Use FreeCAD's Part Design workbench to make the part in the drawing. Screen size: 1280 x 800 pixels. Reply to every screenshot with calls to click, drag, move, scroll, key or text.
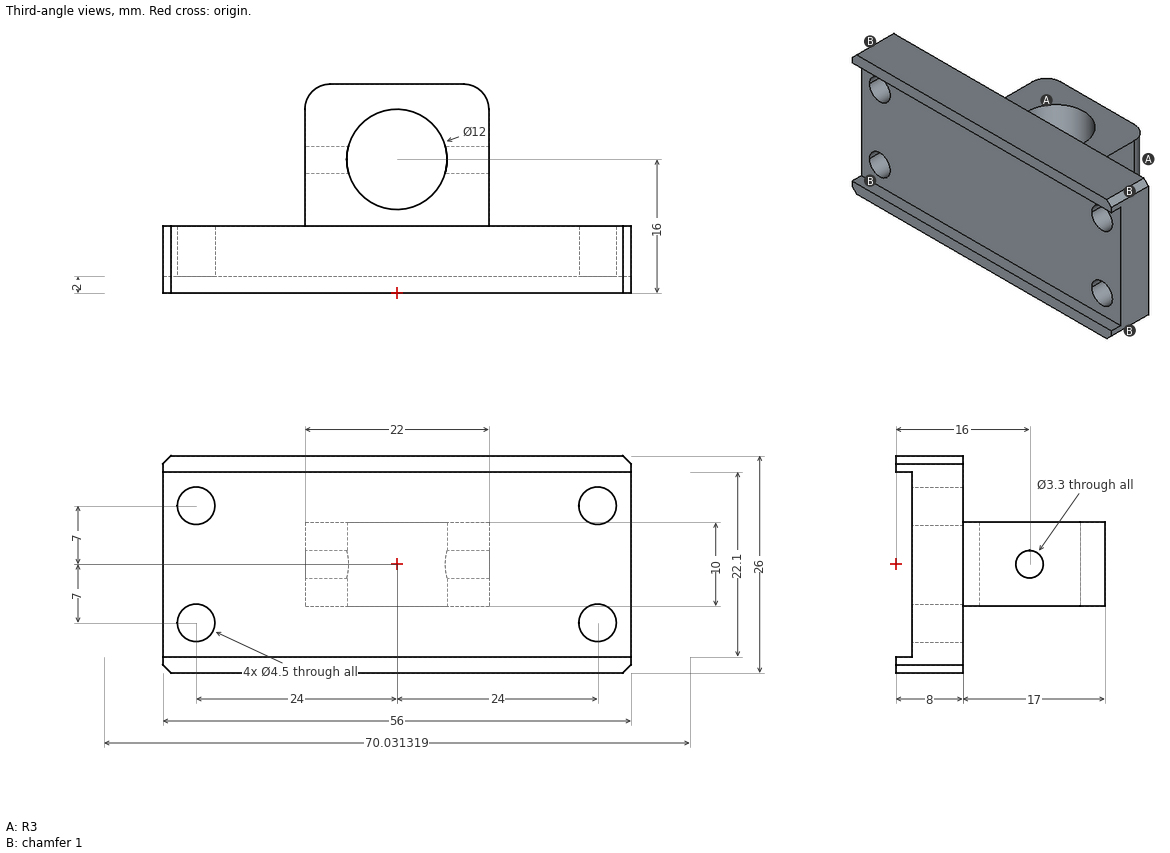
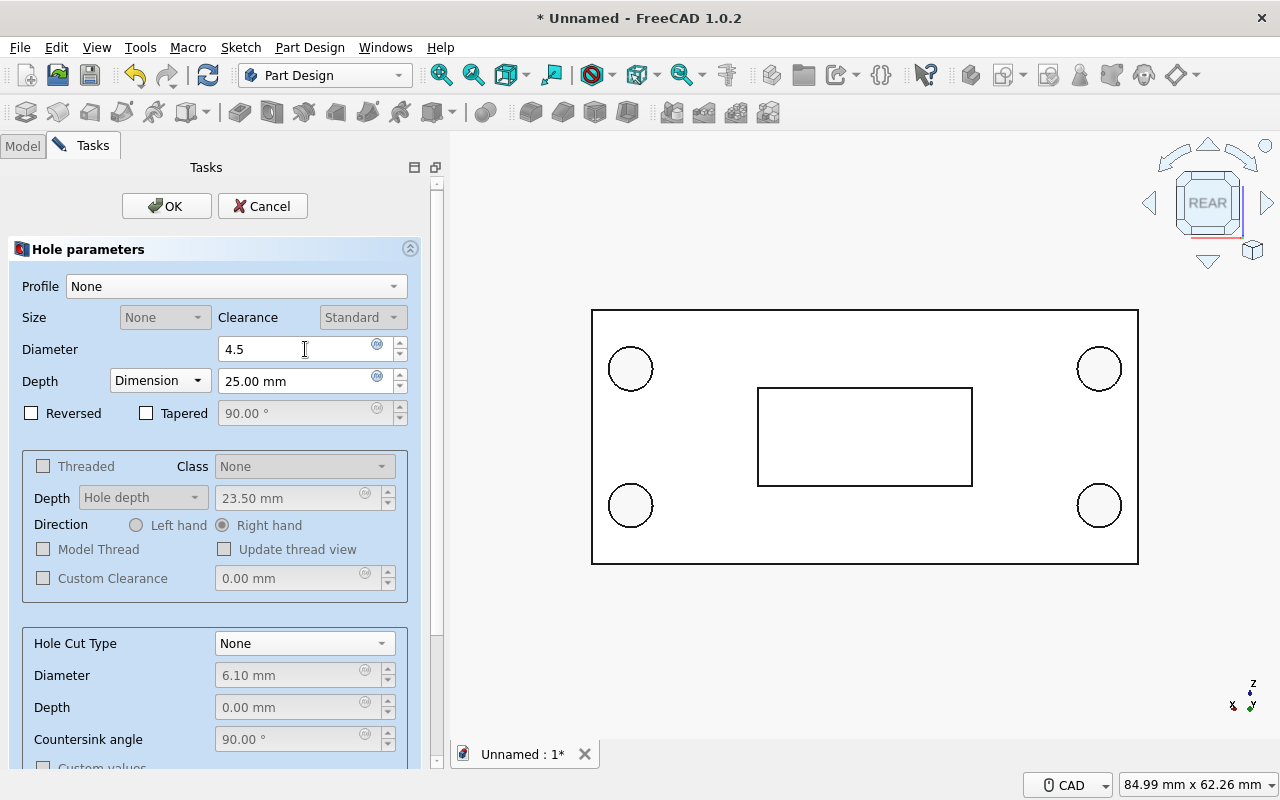
click(161, 380)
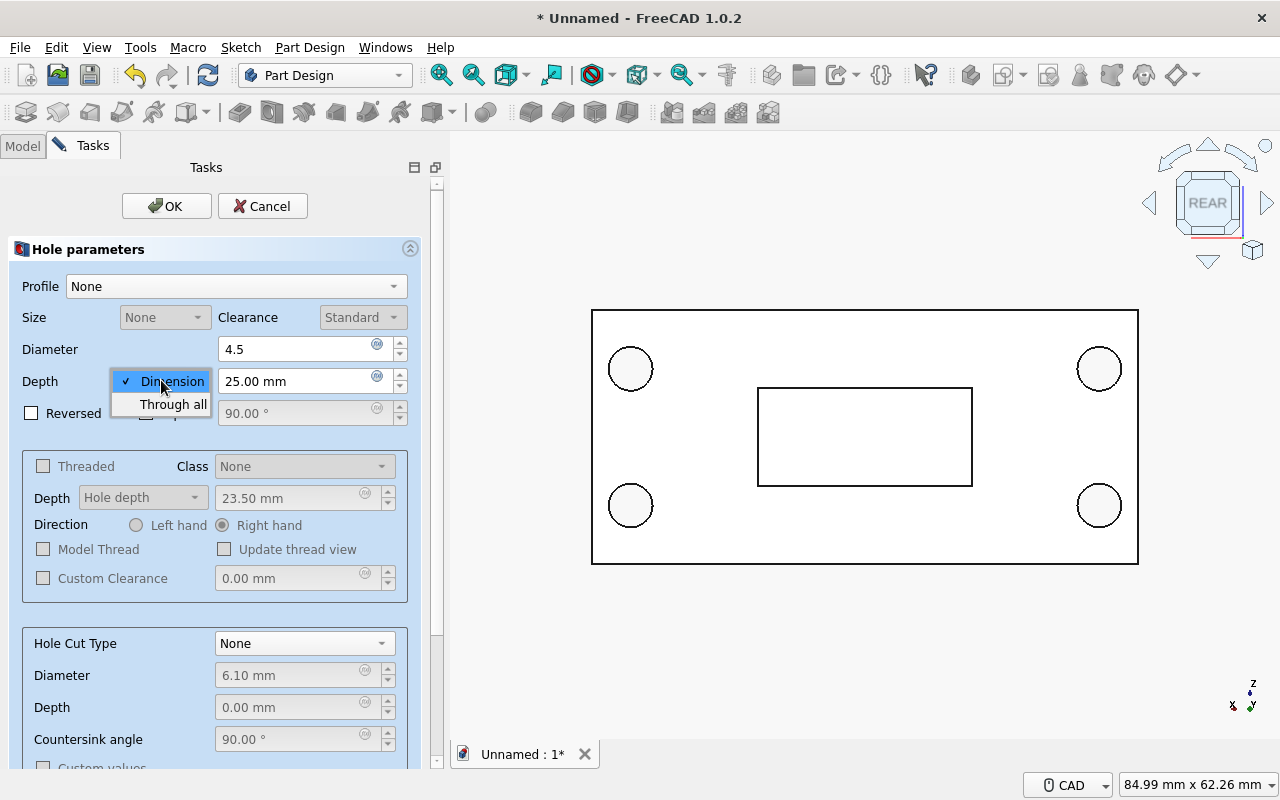
click(160, 404)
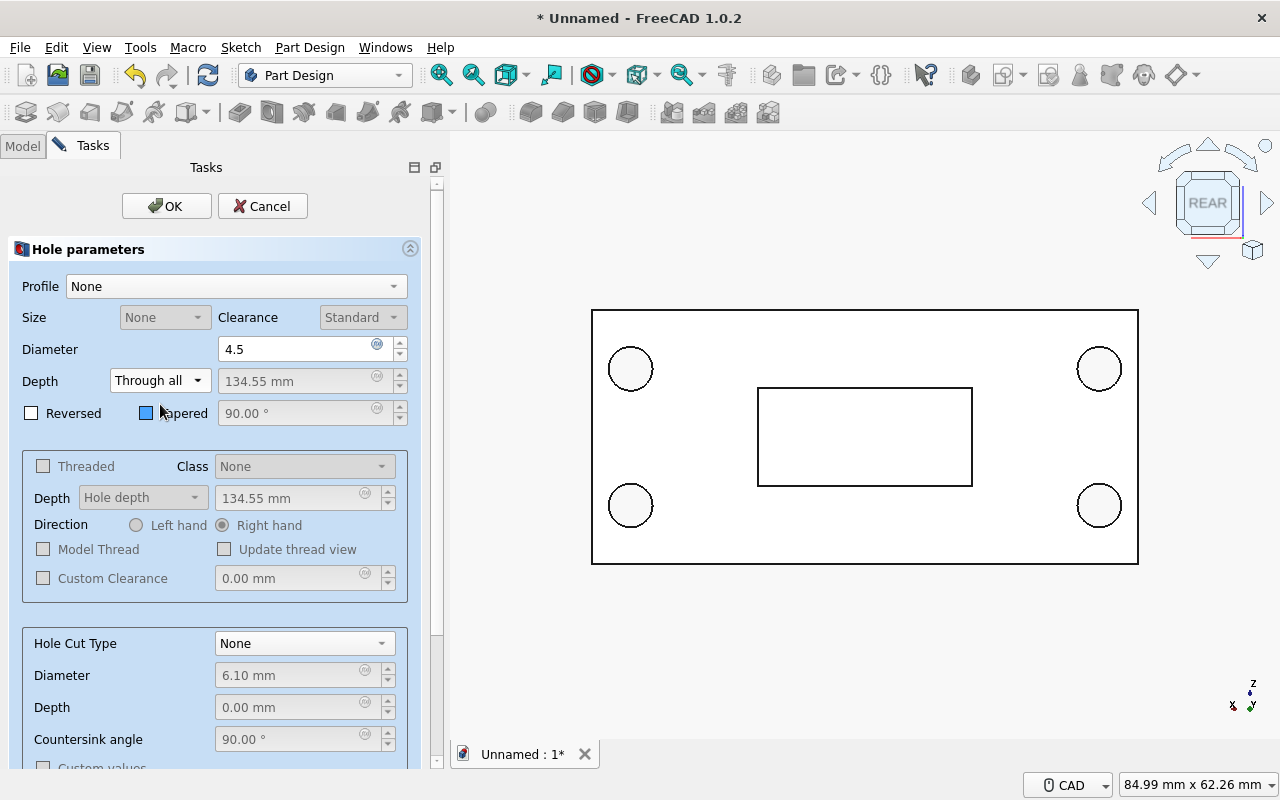
click(167, 206)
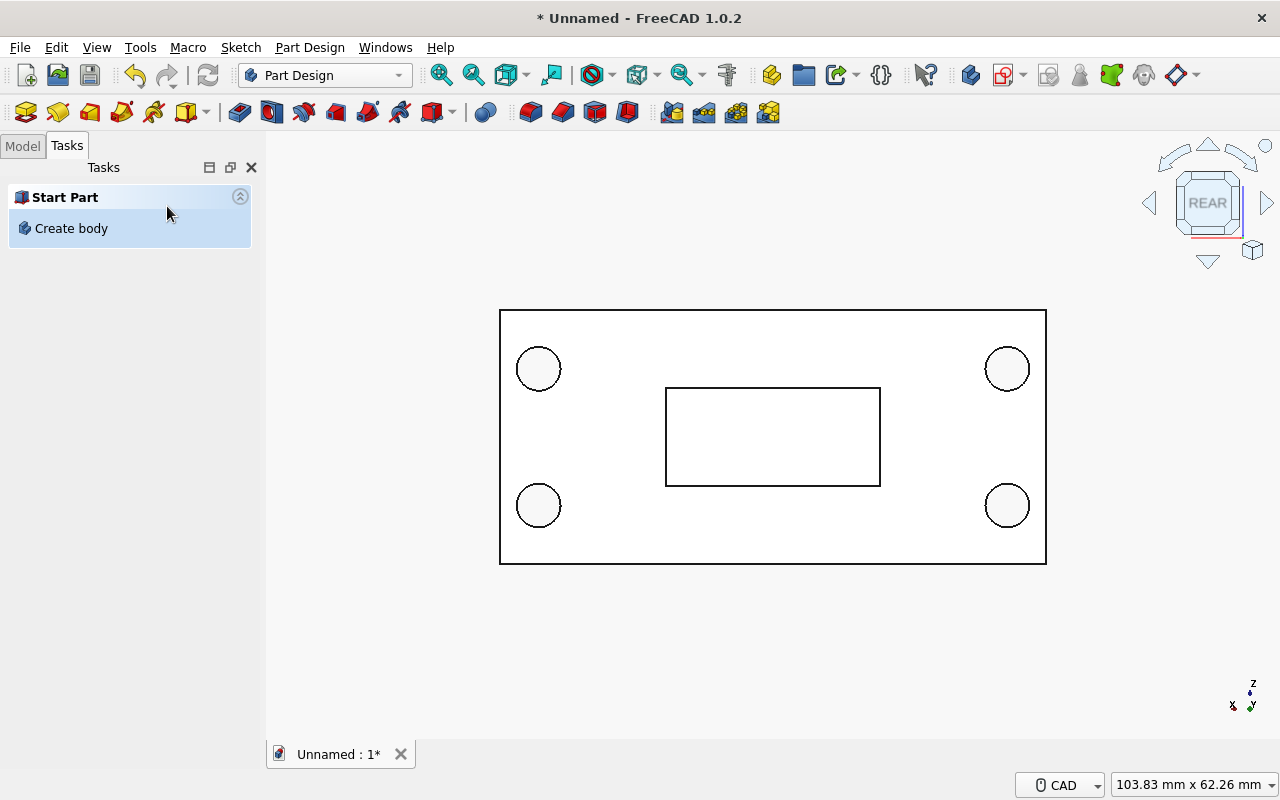
click(880, 436)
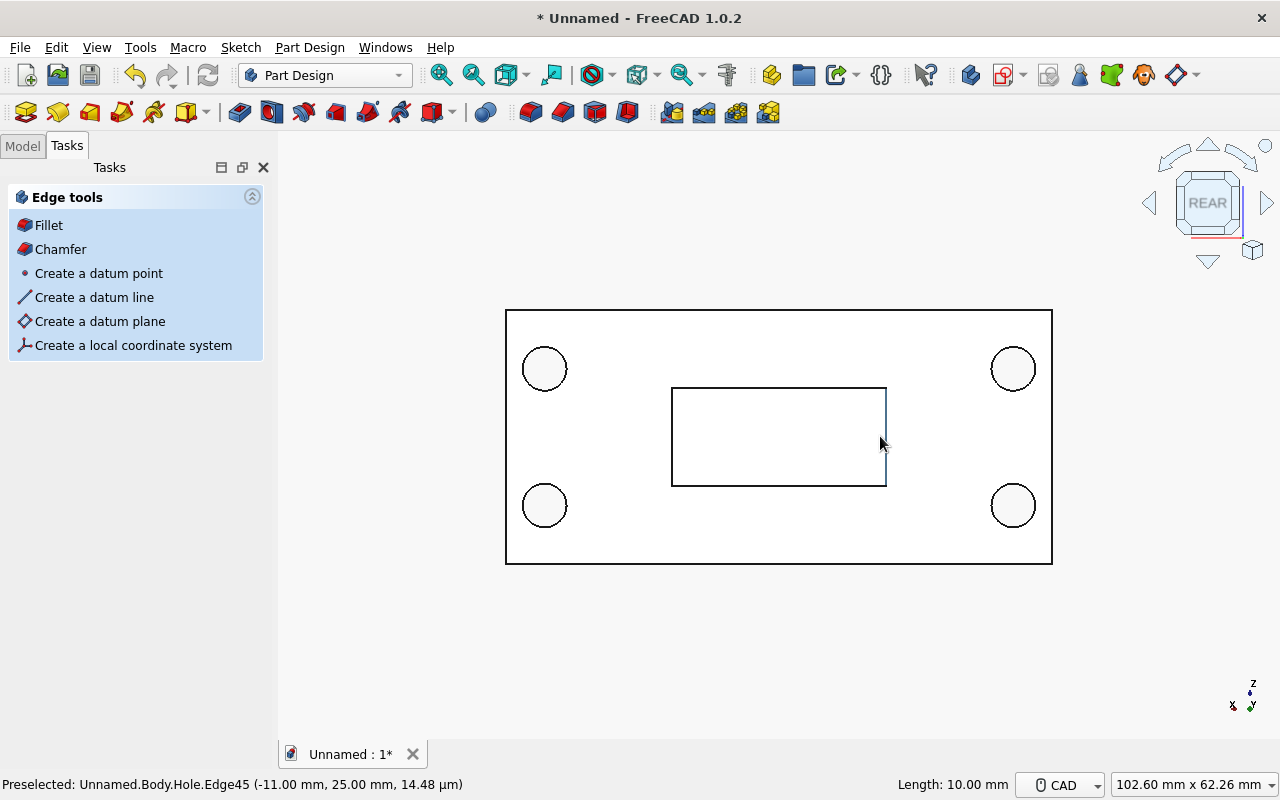
key(0)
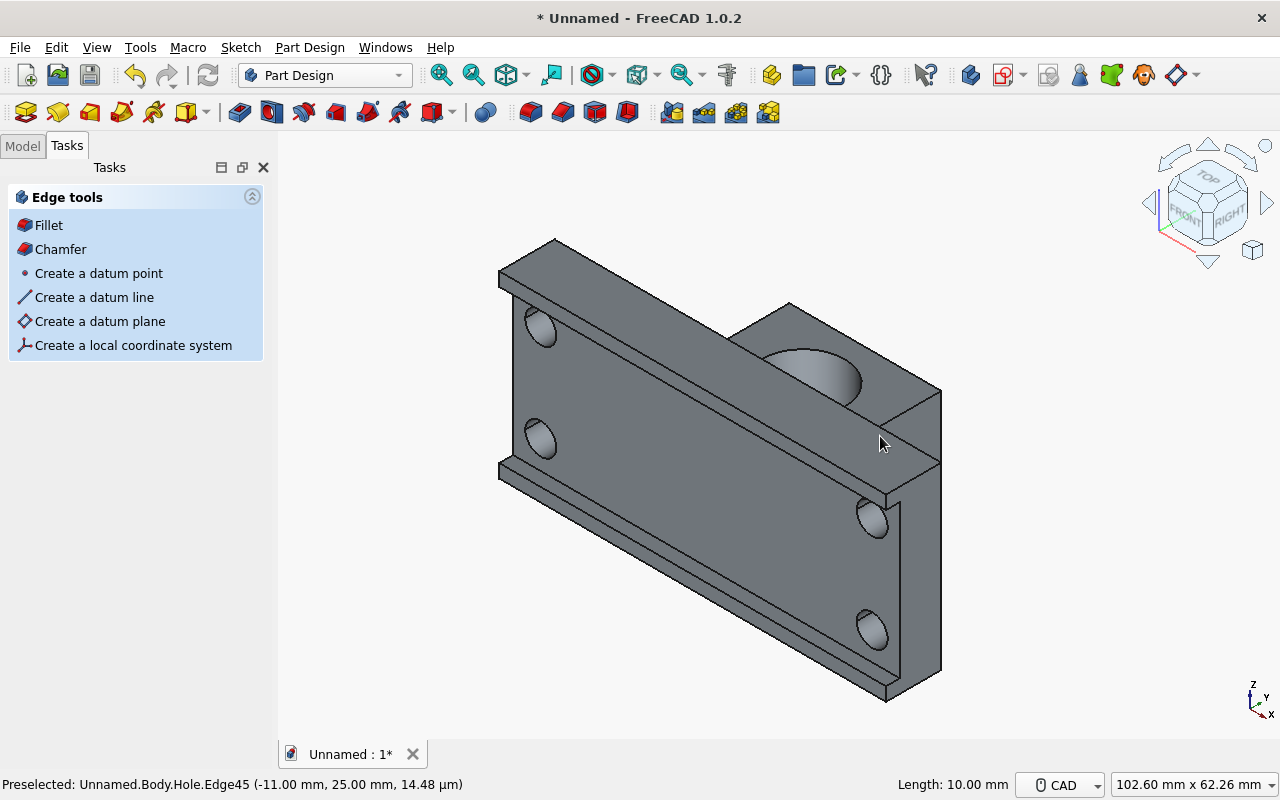
key(2)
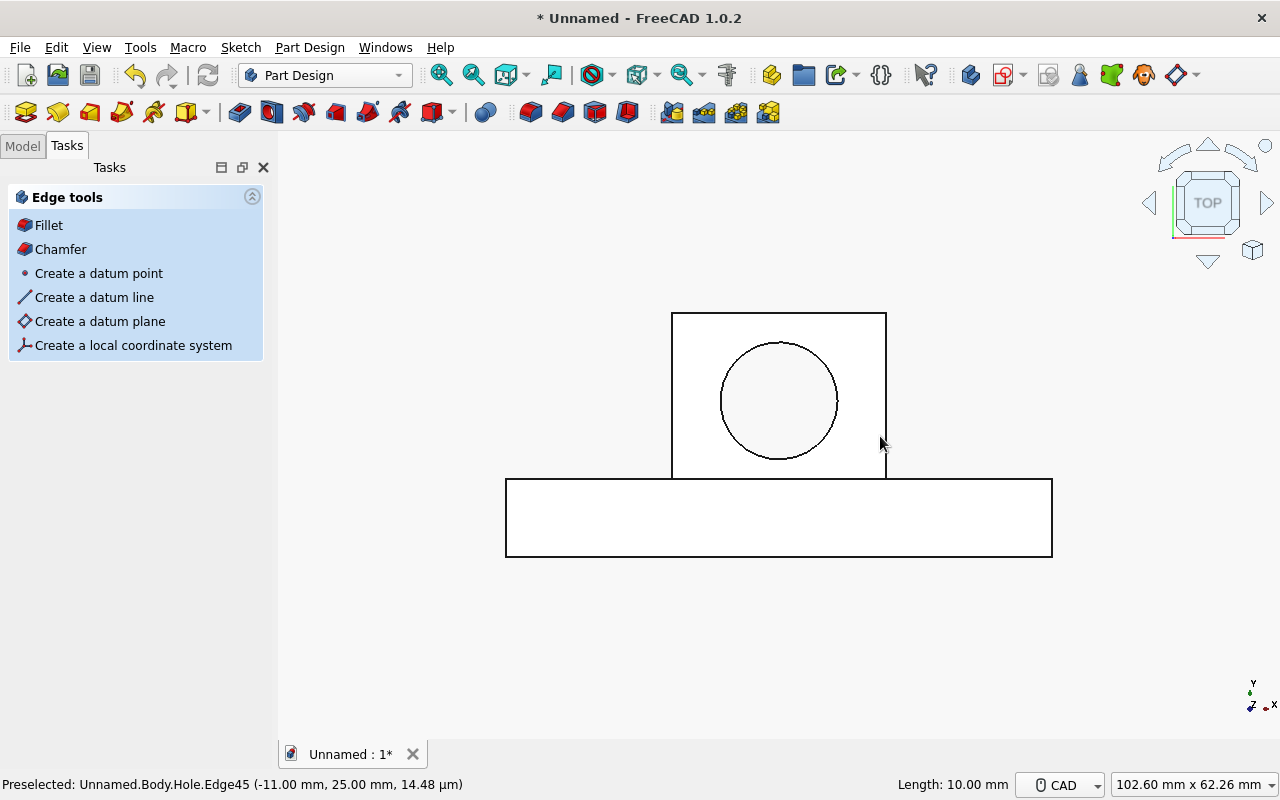
key(1)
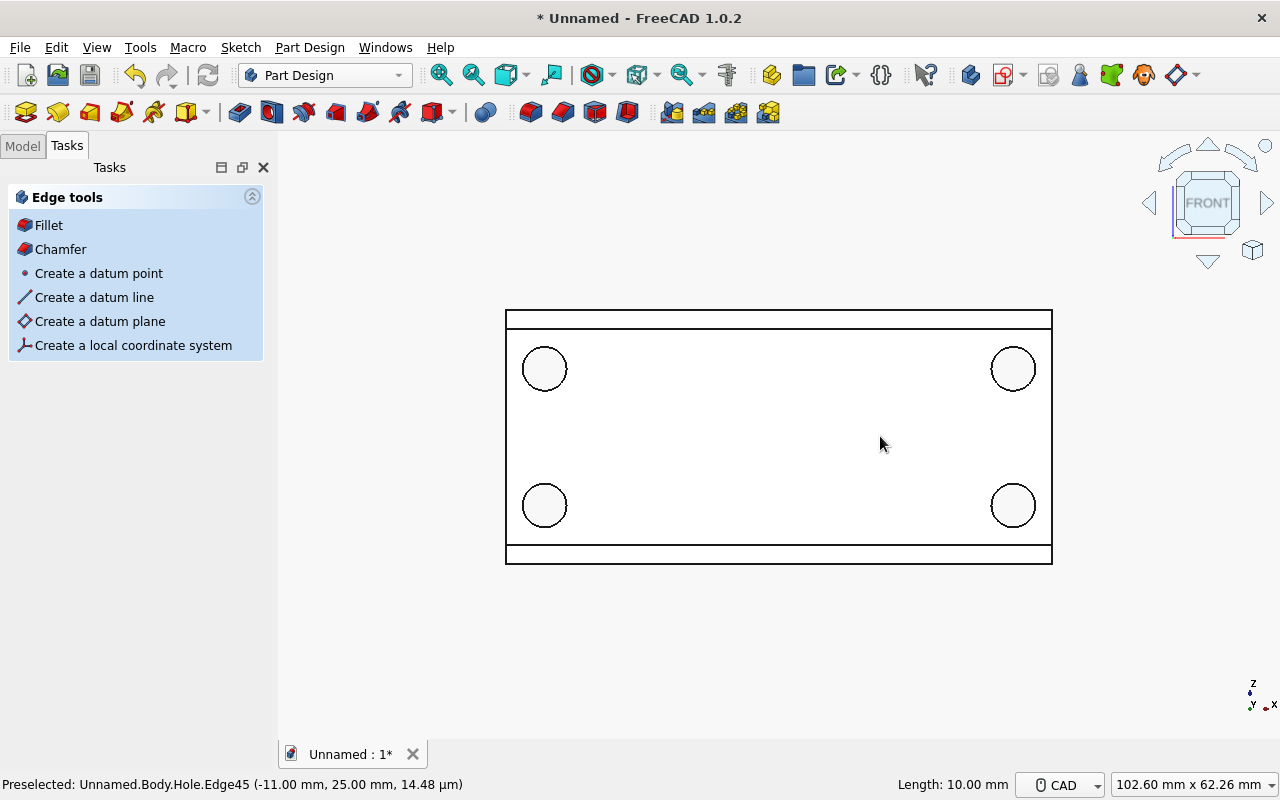
key(3)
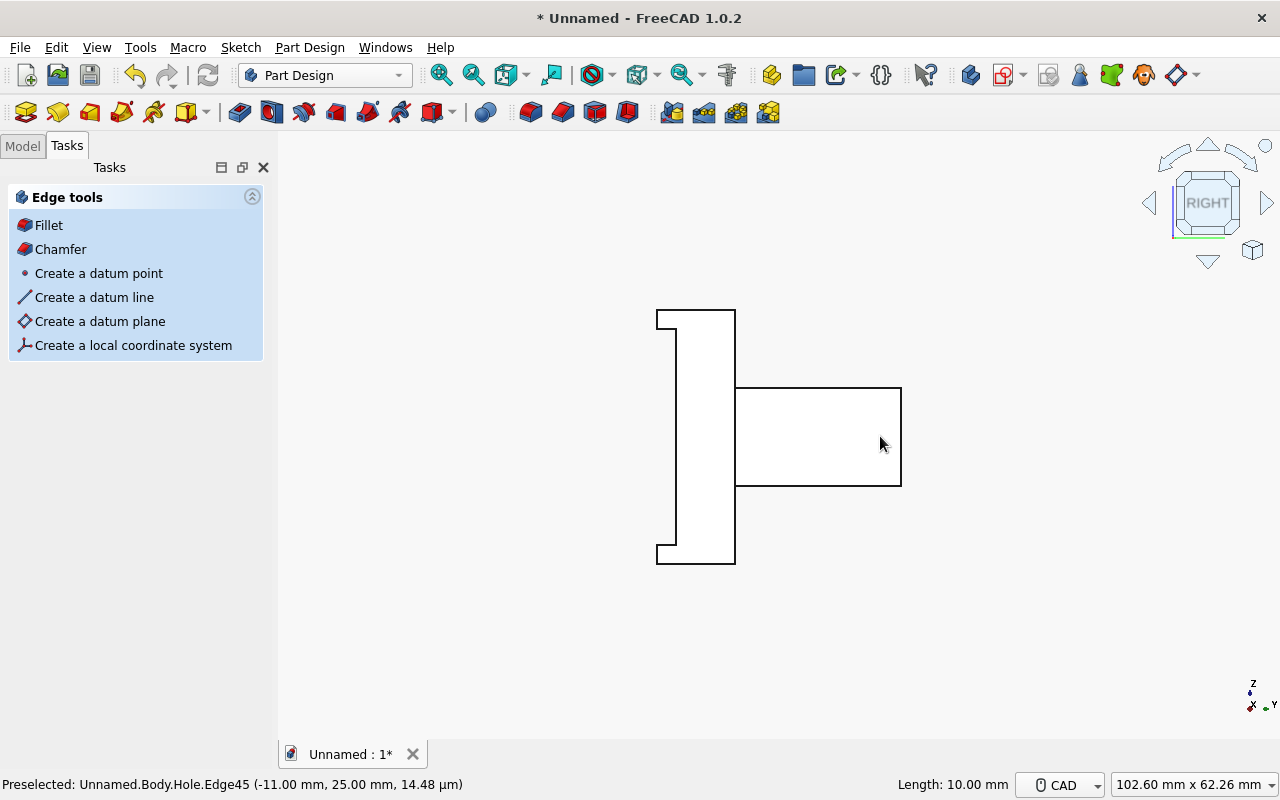
click(442, 76)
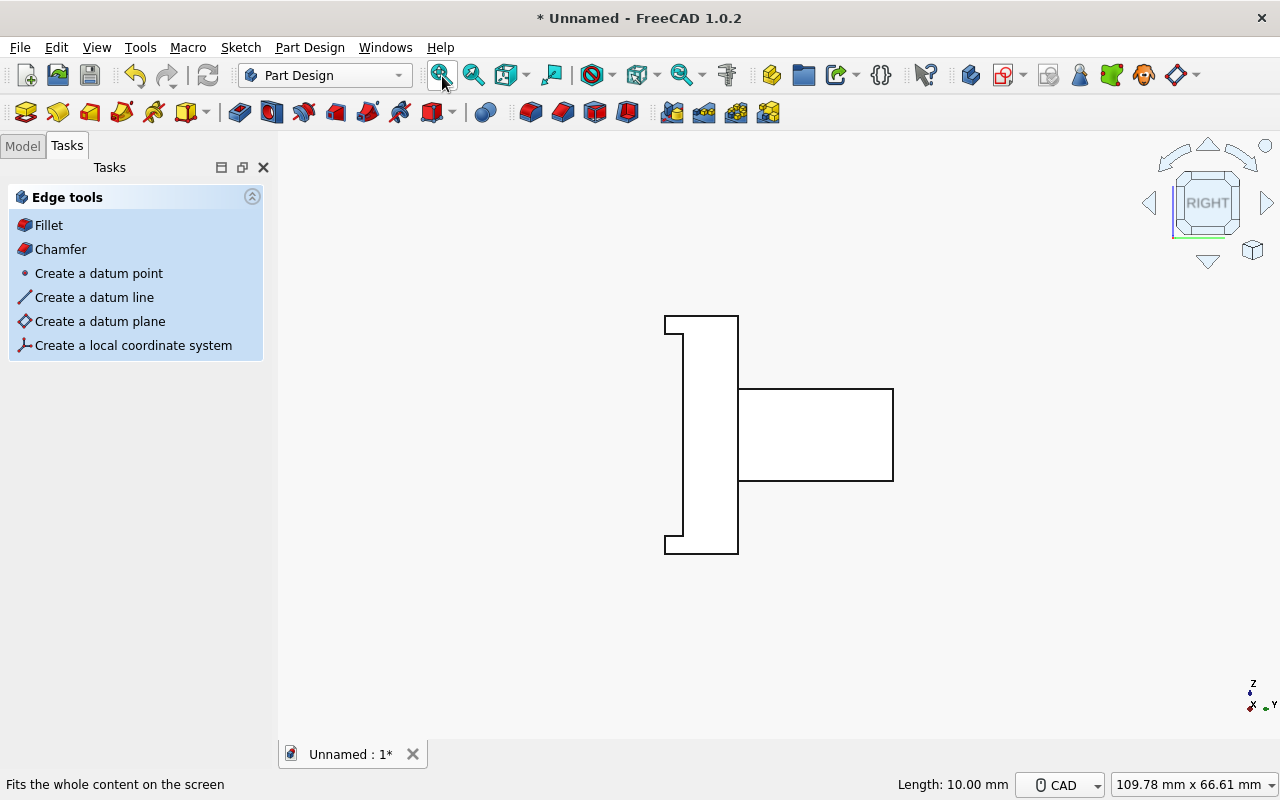
click(893, 434, ctrl)